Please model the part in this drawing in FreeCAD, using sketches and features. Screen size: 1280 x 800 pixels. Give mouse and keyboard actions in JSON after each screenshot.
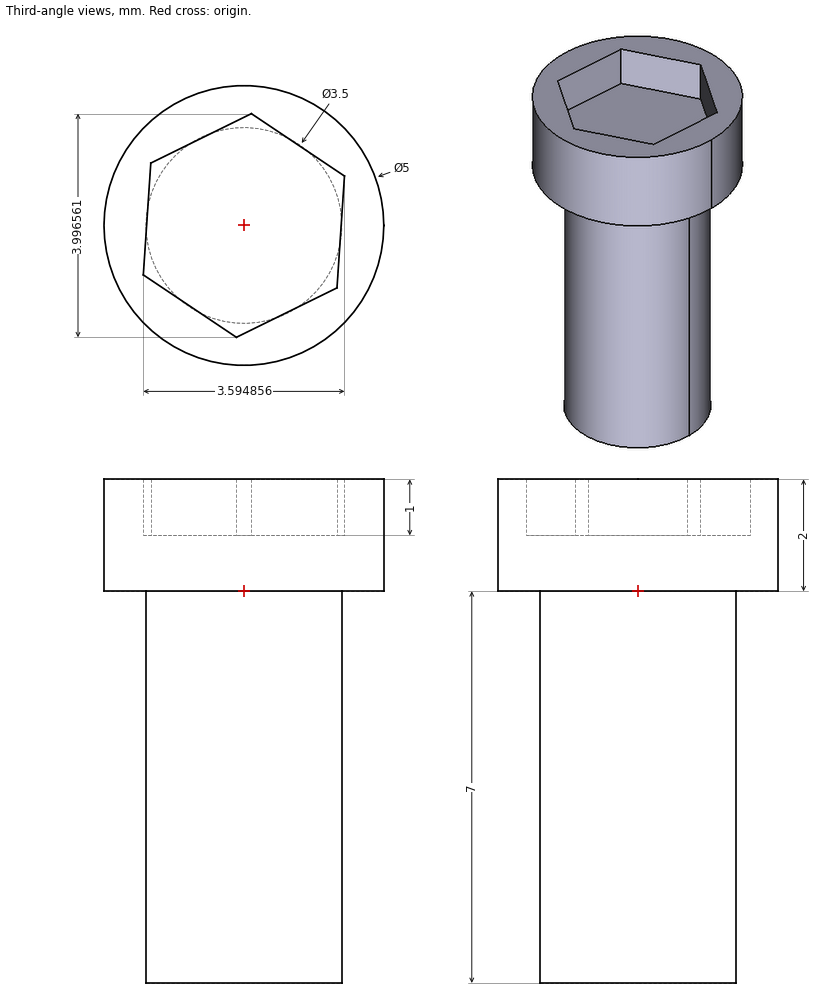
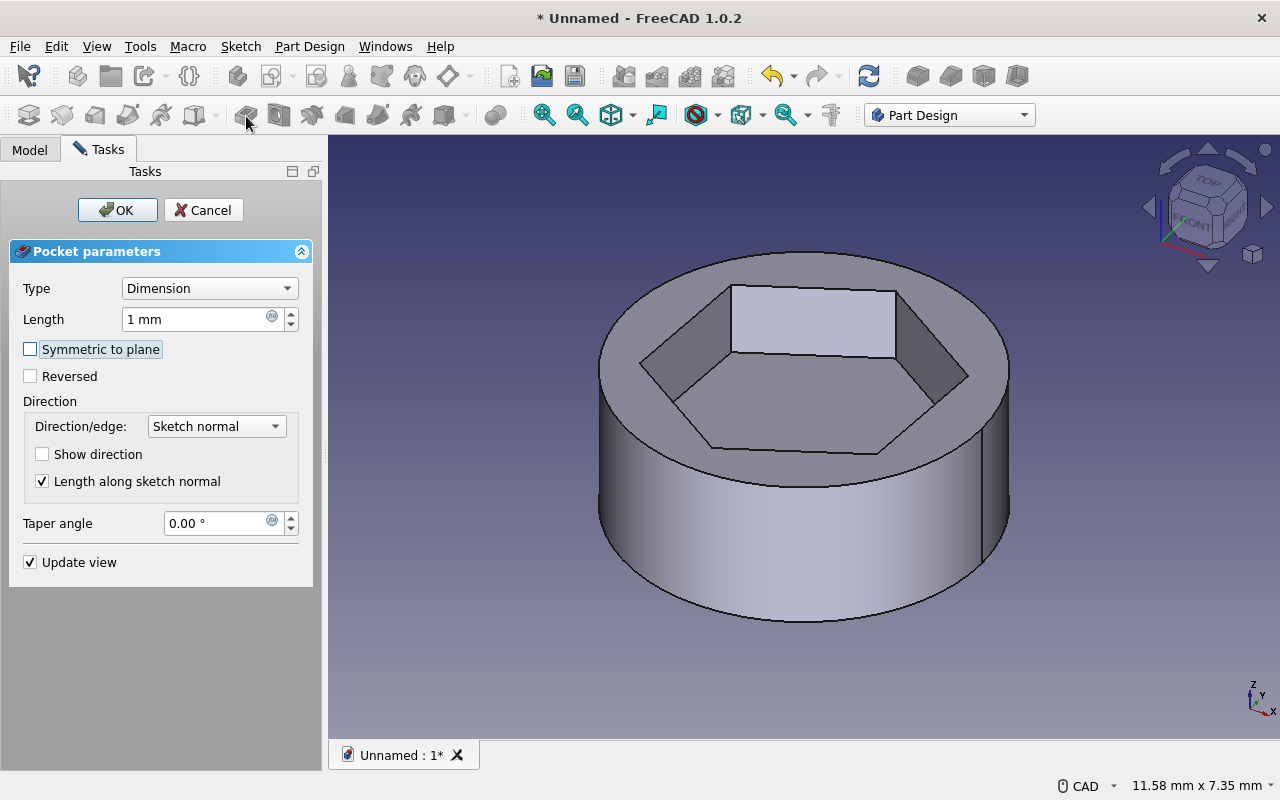
{"action": "left_click", "coordinate": [118, 210]}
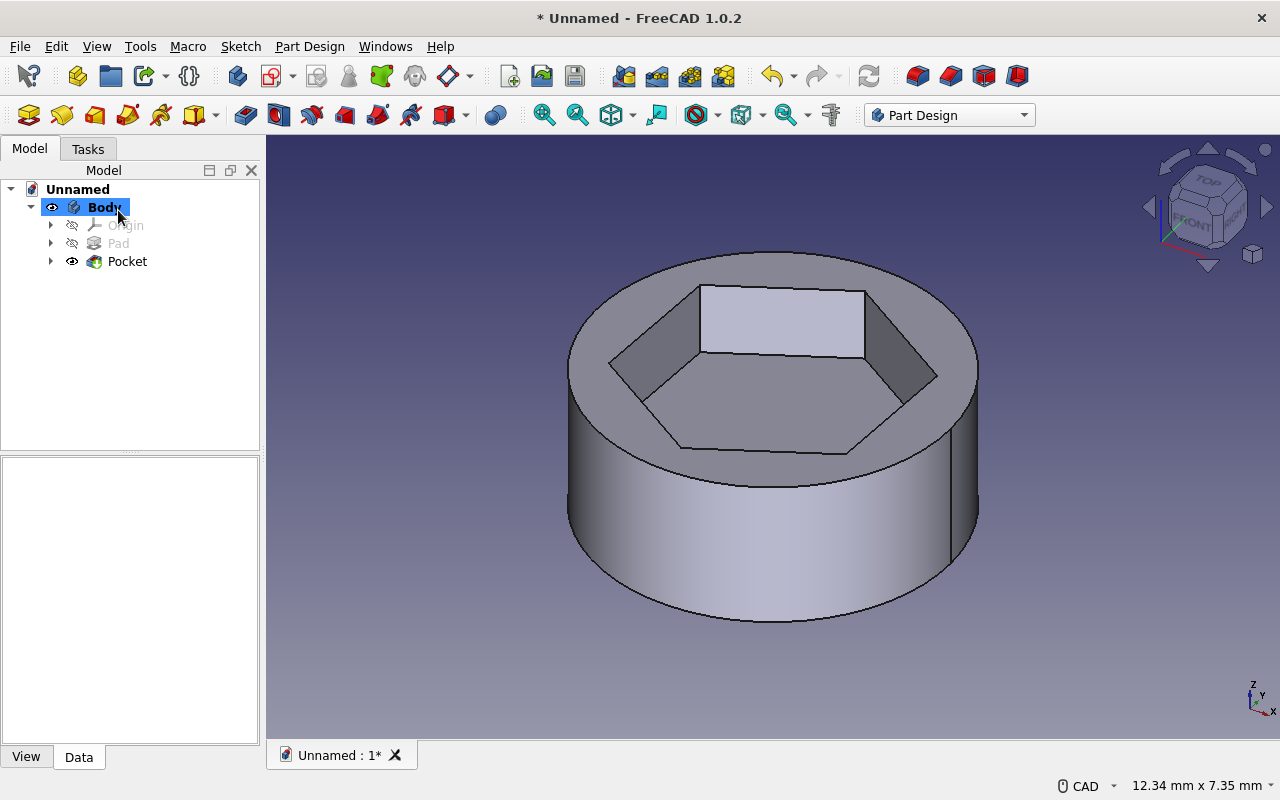
{"action": "key", "text": "5"}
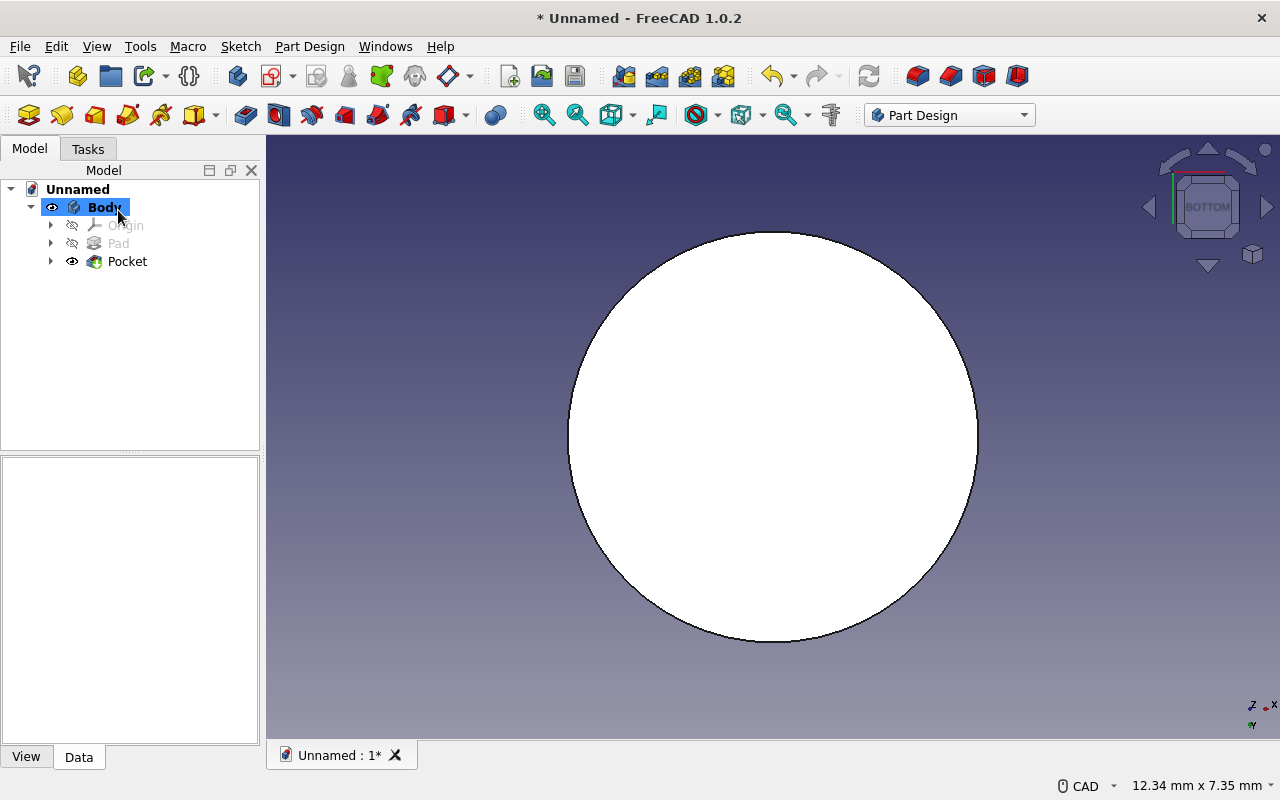
{"action": "left_click", "coordinate": [773, 436]}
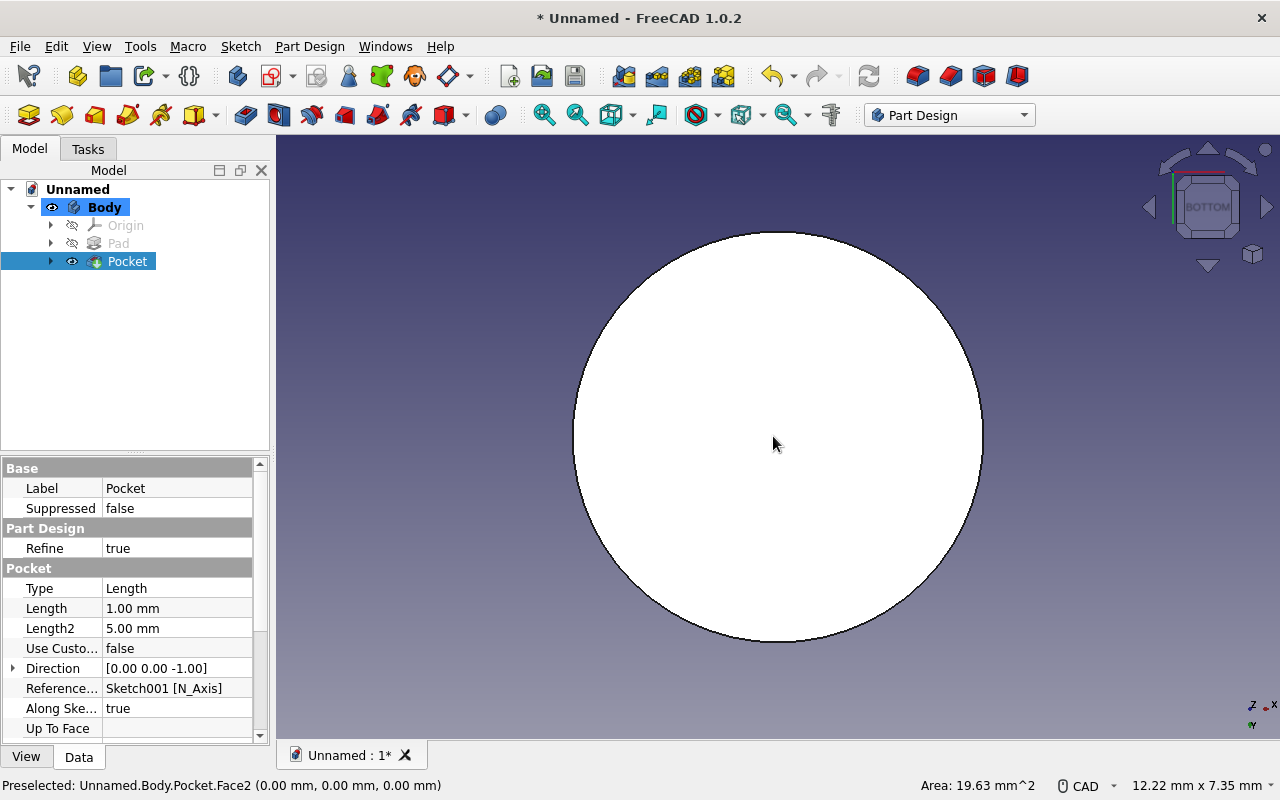
{"action": "left_click", "coordinate": [270, 76]}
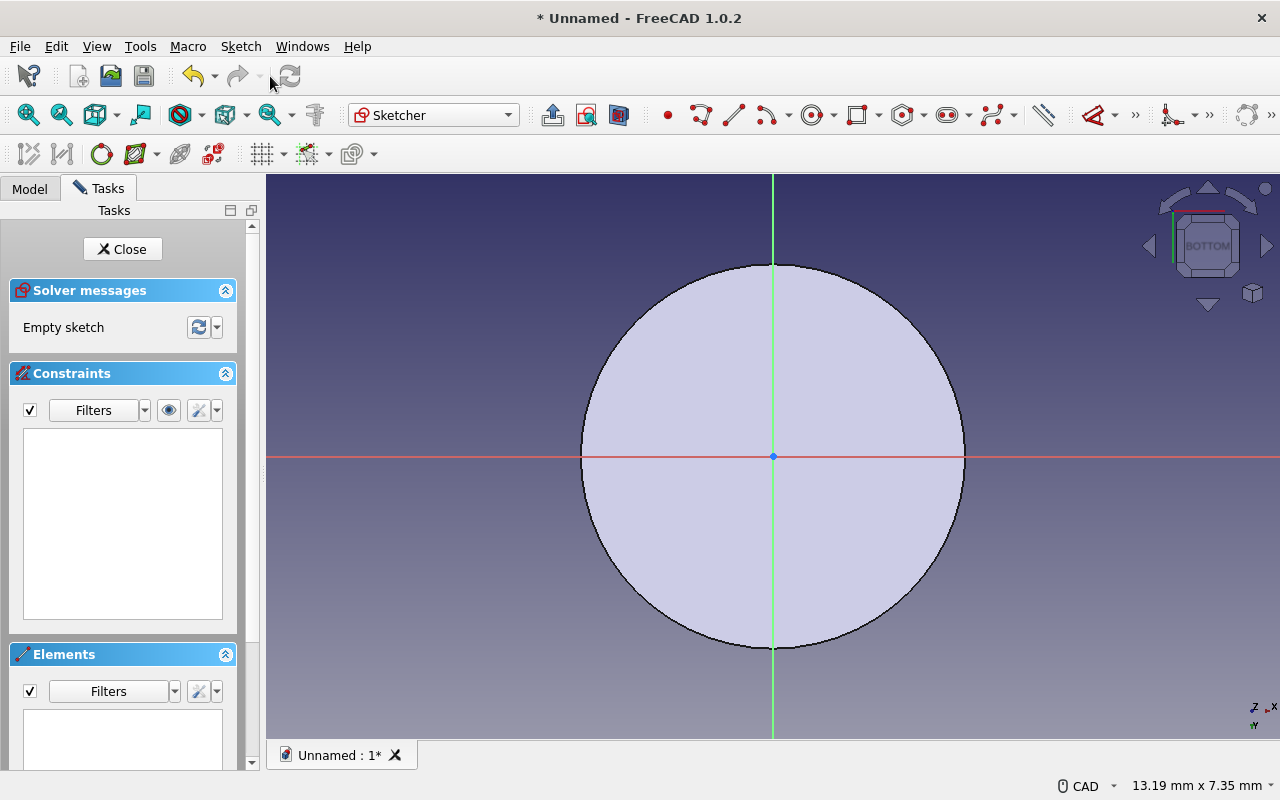
{"action": "left_click", "coordinate": [812, 116]}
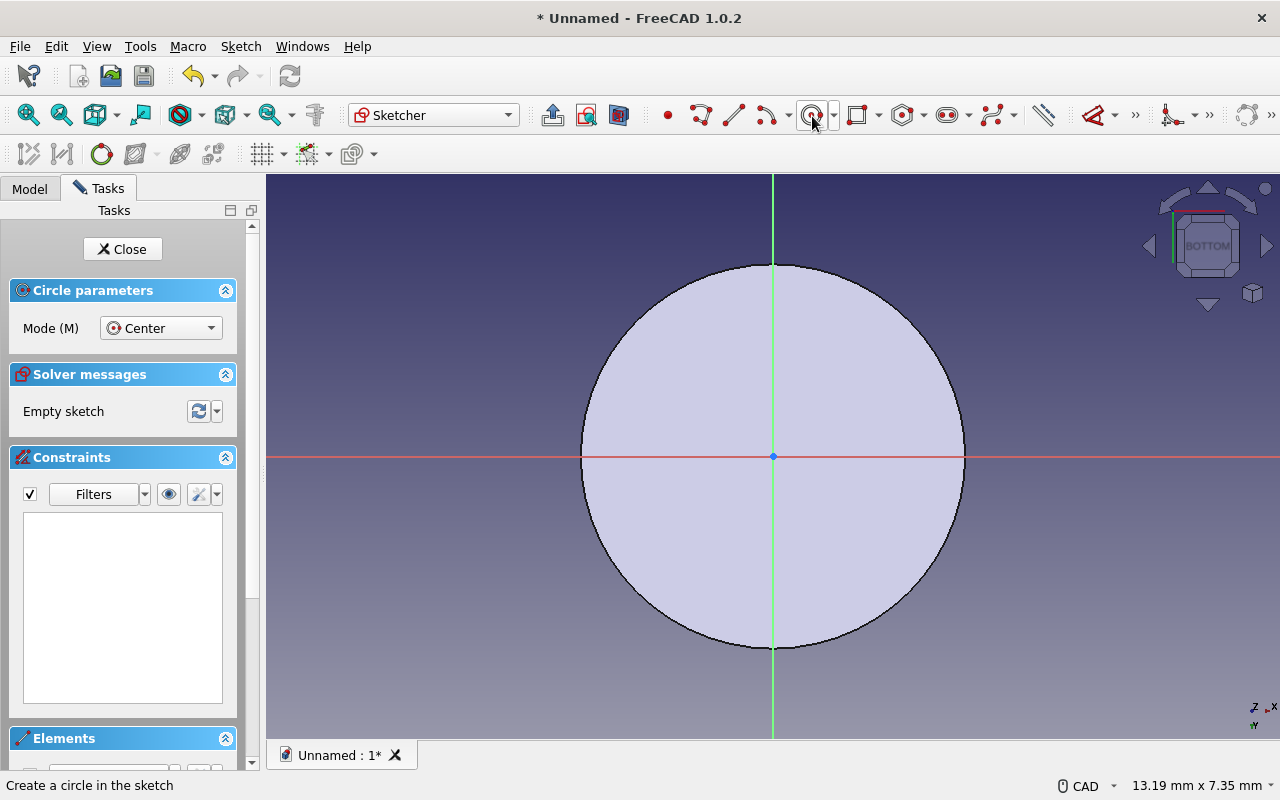
{"action": "left_click", "coordinate": [773, 456]}
{"action": "left_click", "coordinate": [868, 361]}
{"action": "key", "text": "Escape"}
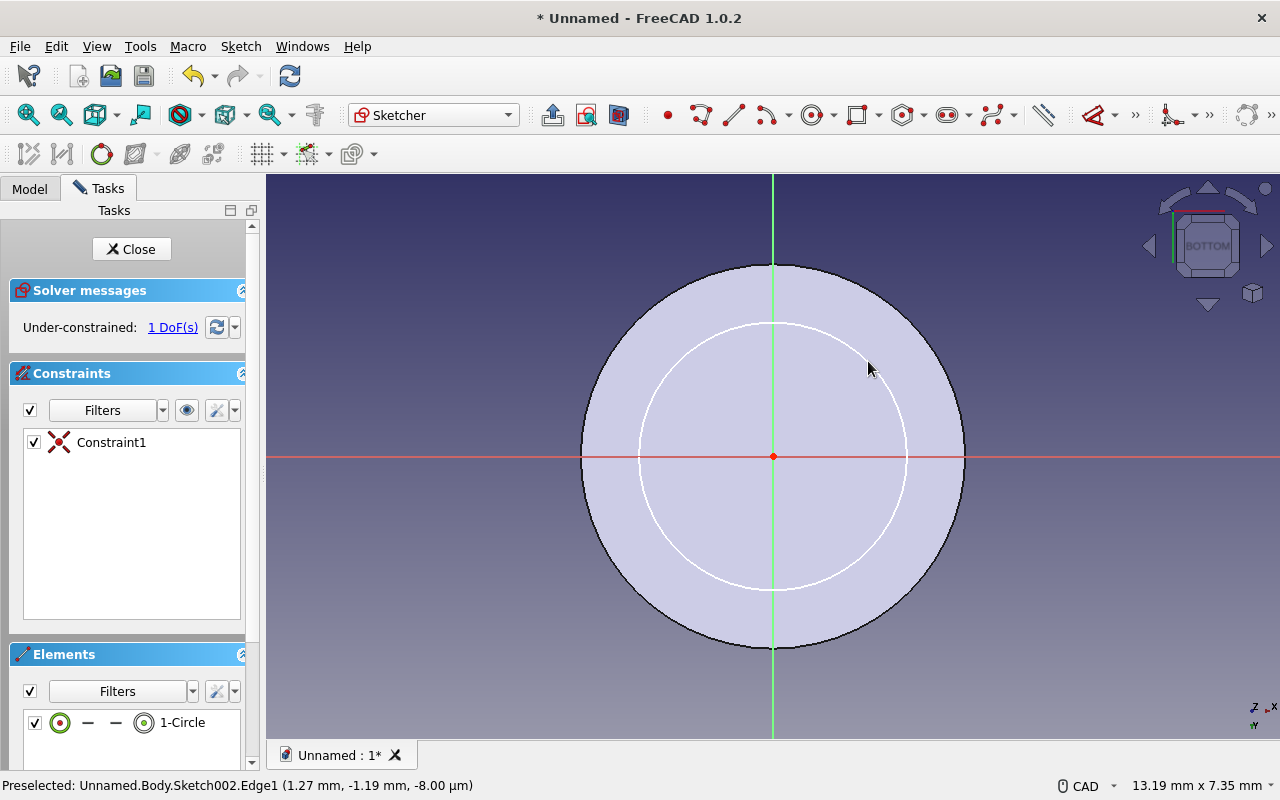
{"action": "left_click", "coordinate": [1092, 116]}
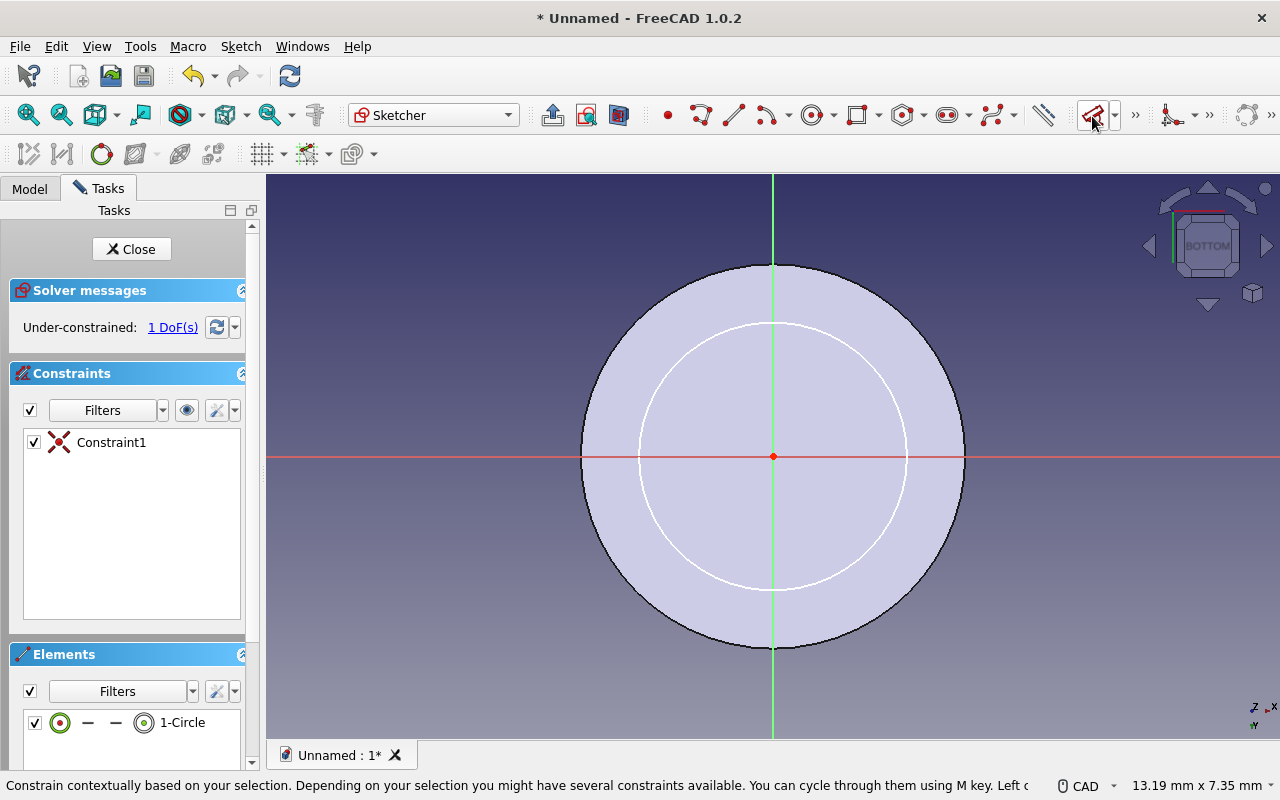
{"action": "left_click", "coordinate": [867, 361]}
{"action": "left_click", "coordinate": [889, 338]}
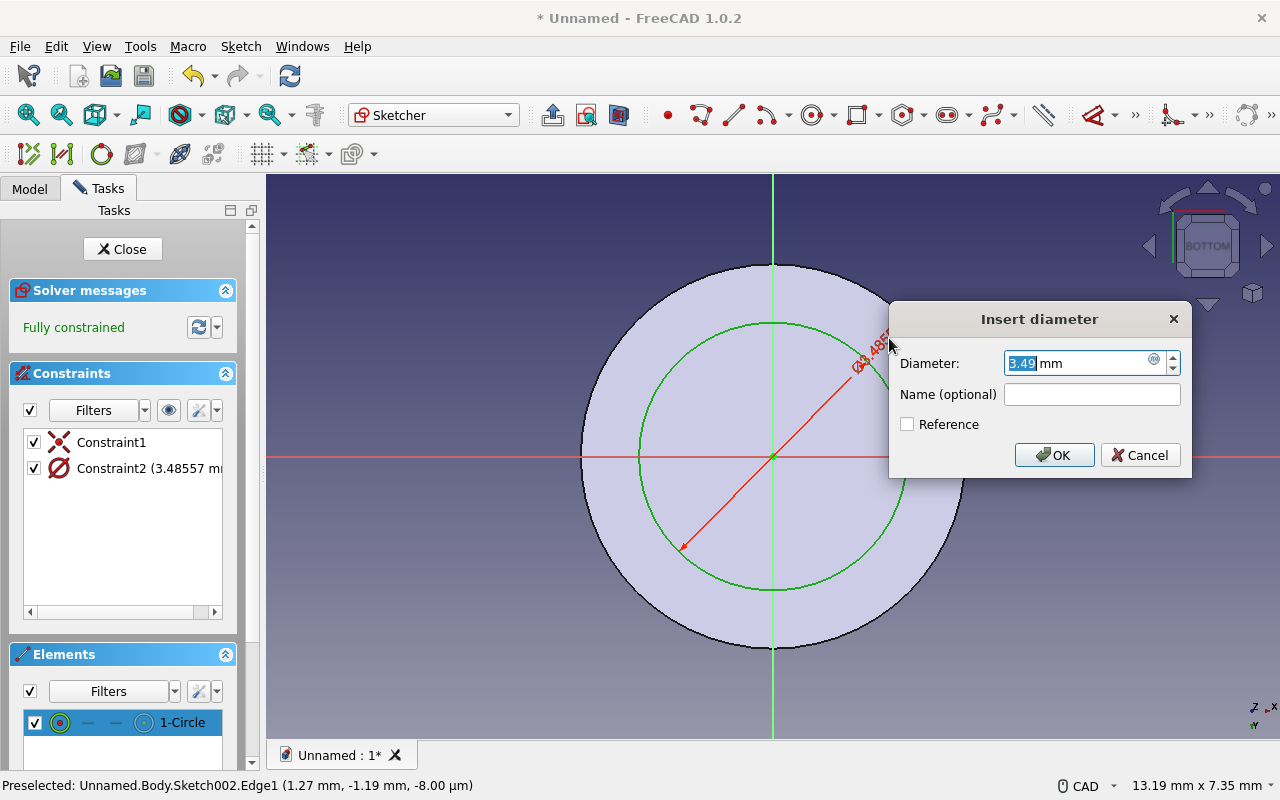
{"action": "type", "text": "3.5"}
{"action": "key", "text": "Return"}
{"action": "key", "text": "Escape"}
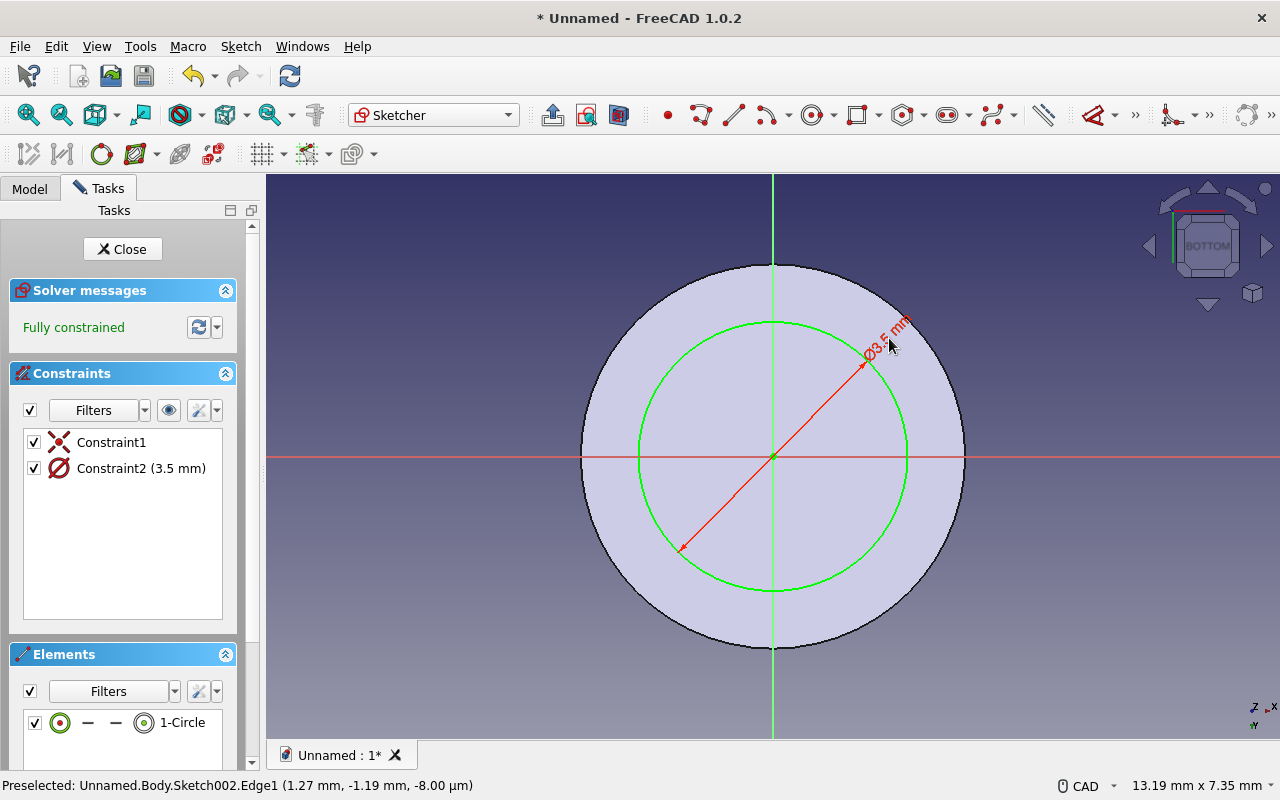
{"action": "left_click", "coordinate": [123, 249]}